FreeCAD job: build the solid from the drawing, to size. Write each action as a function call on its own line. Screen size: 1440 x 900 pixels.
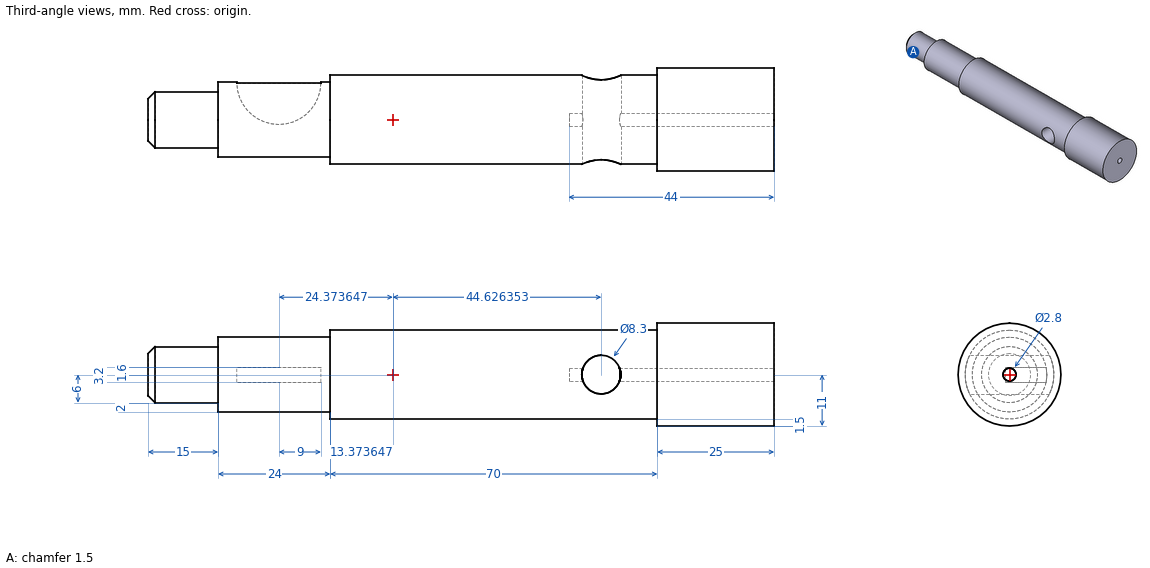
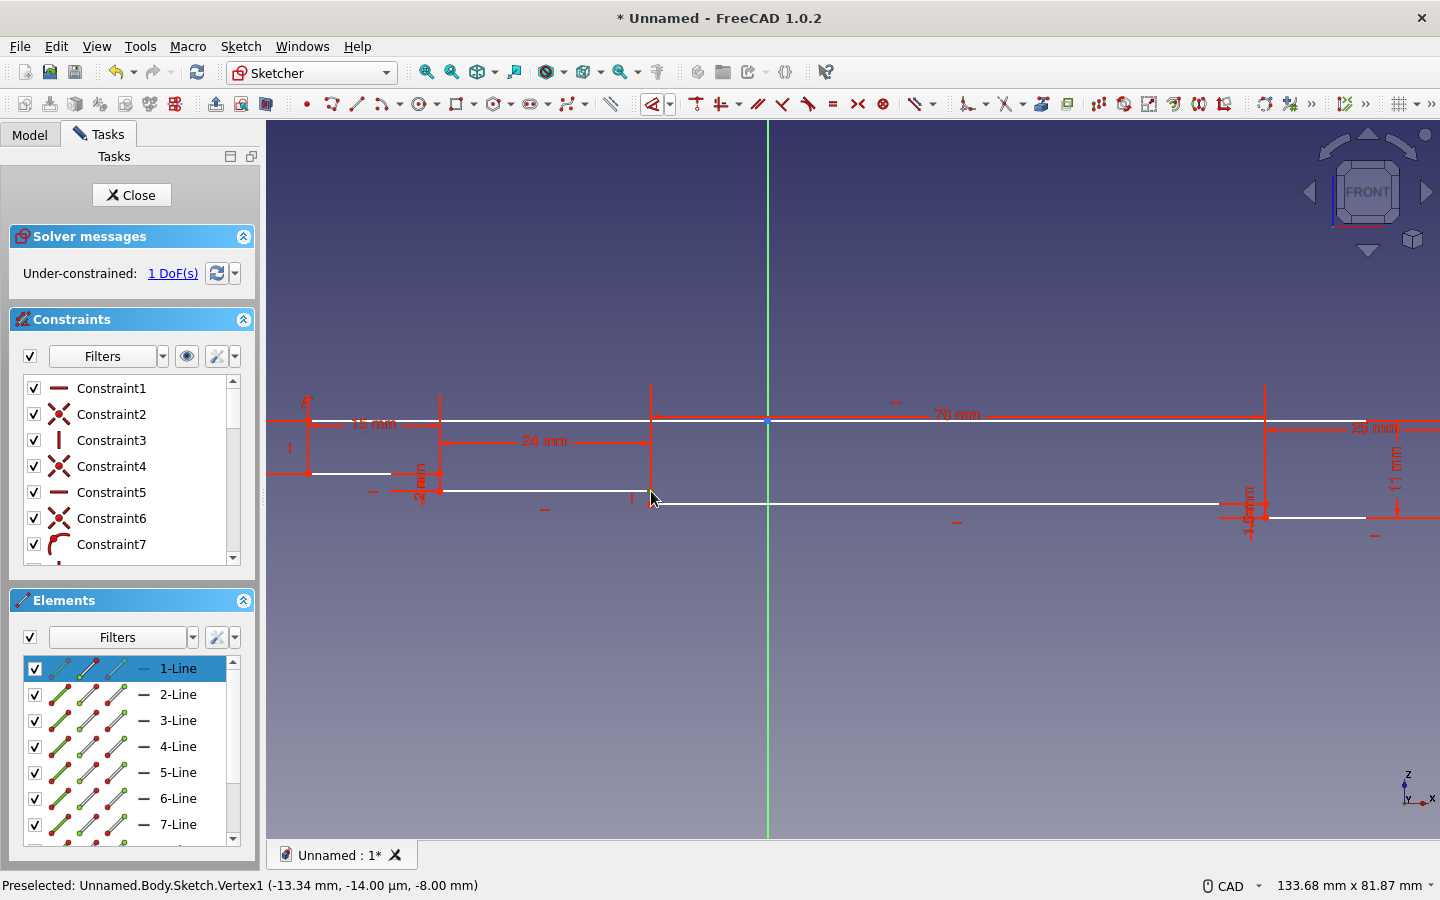
click(670, 104)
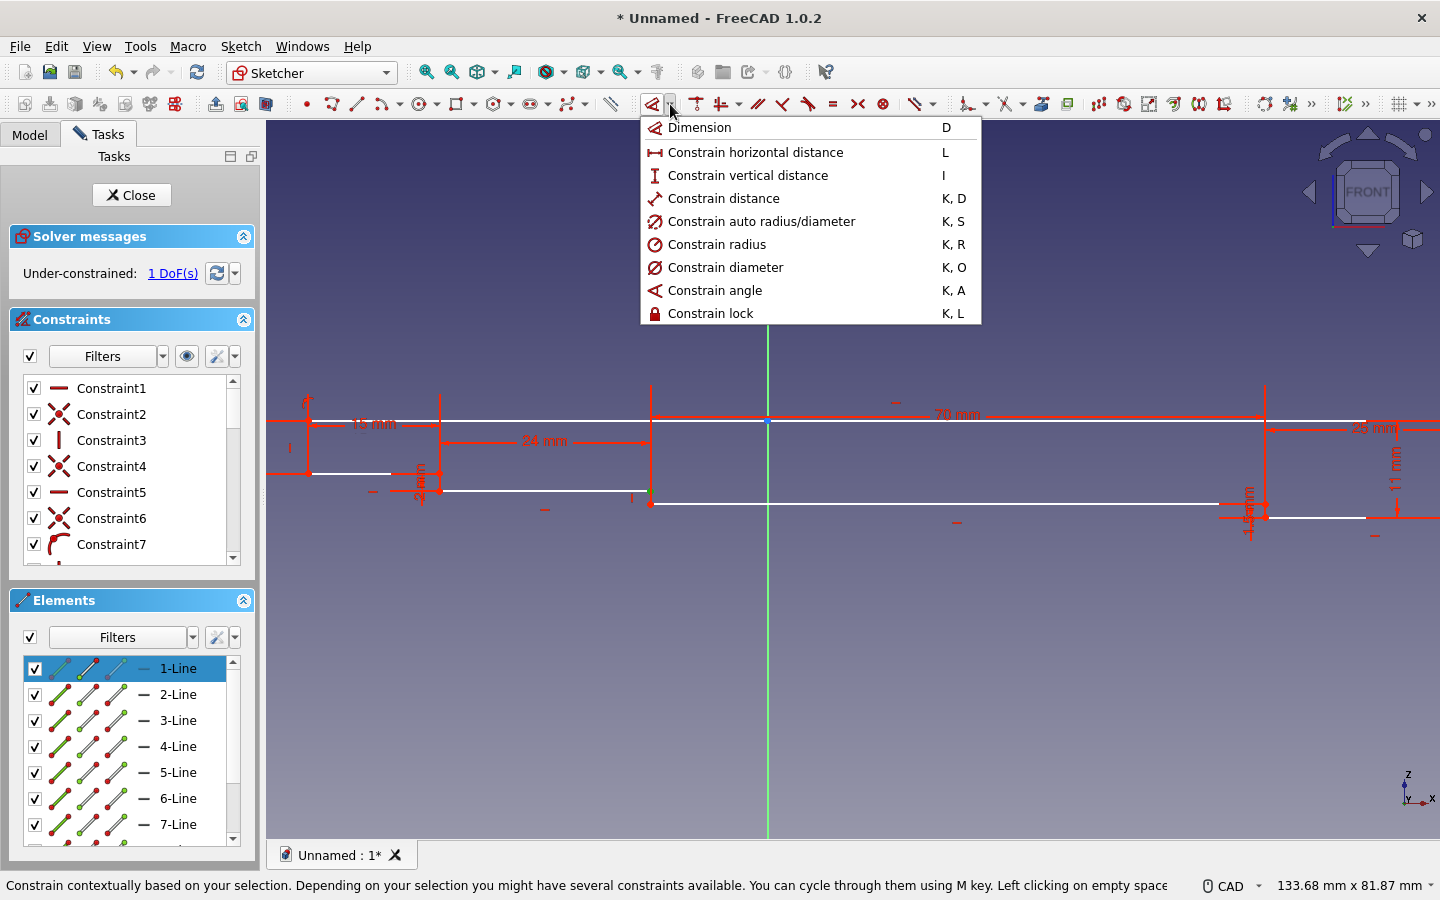
click(811, 152)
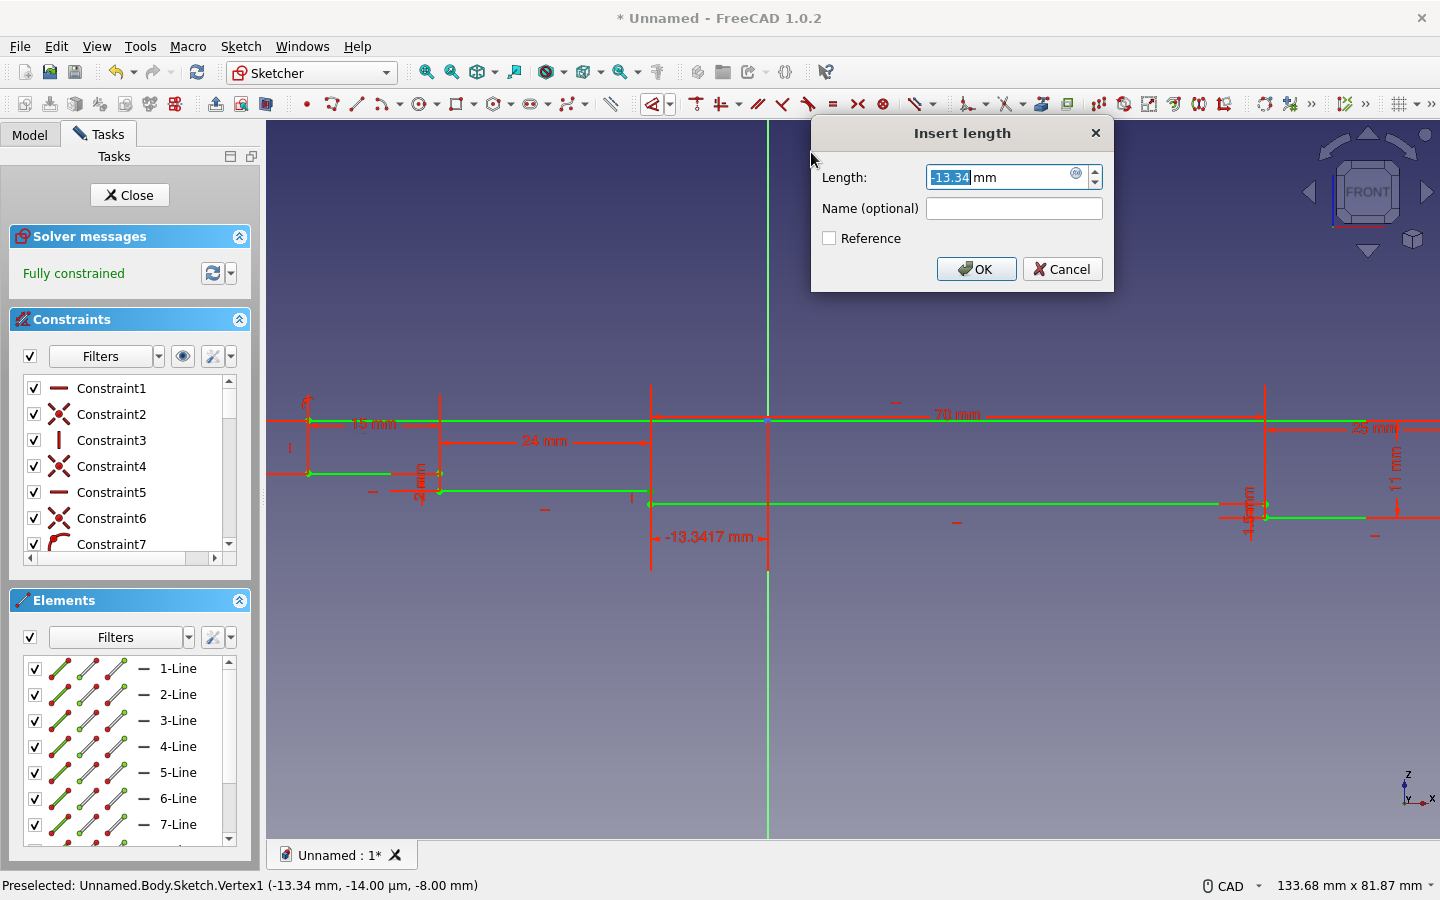
text(-13.373647)
key(Return)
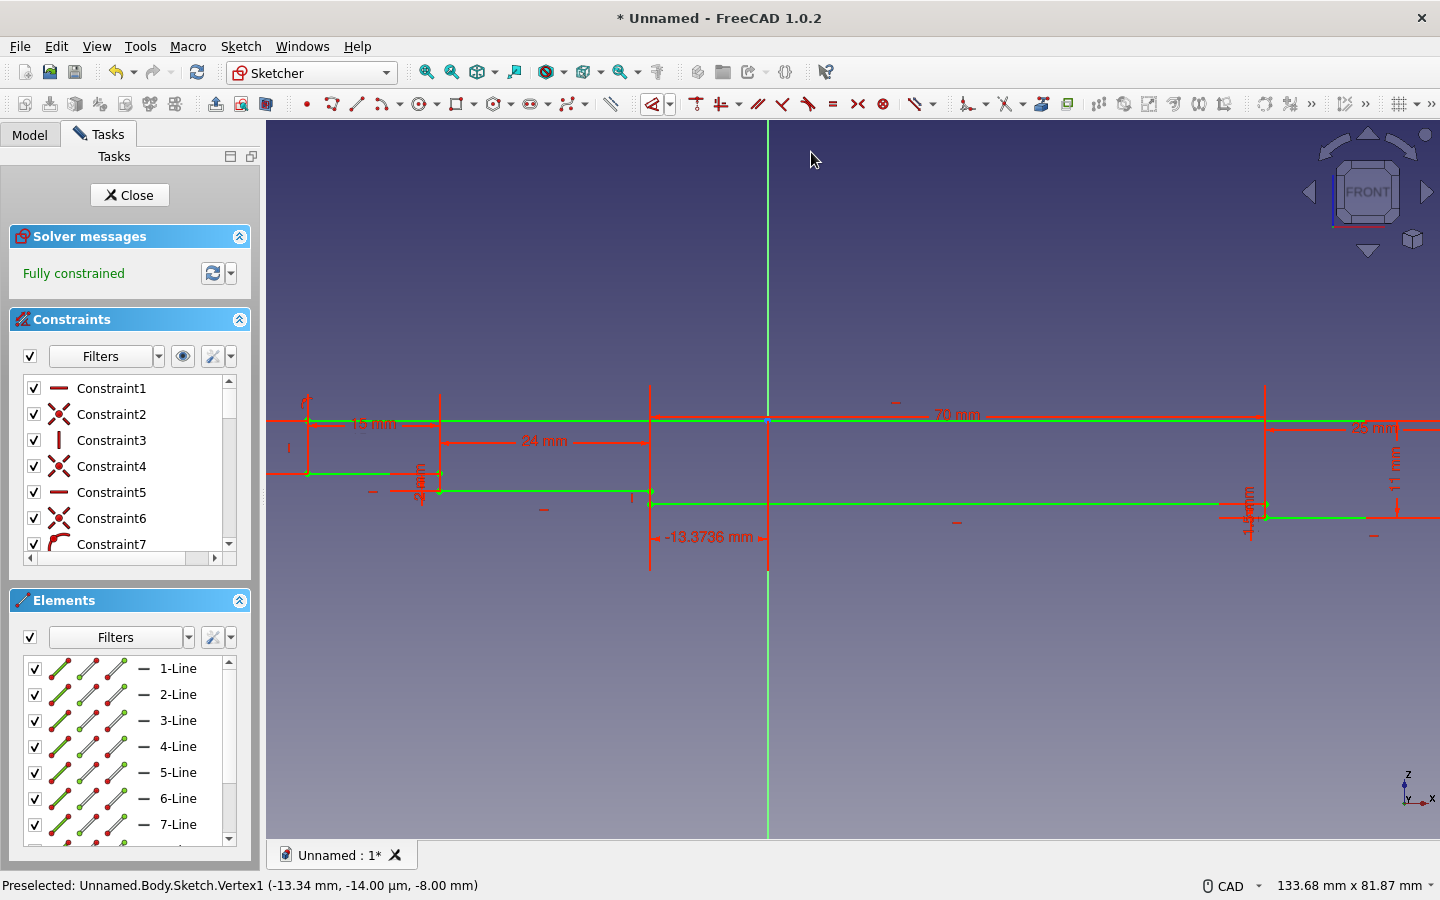
click(130, 195)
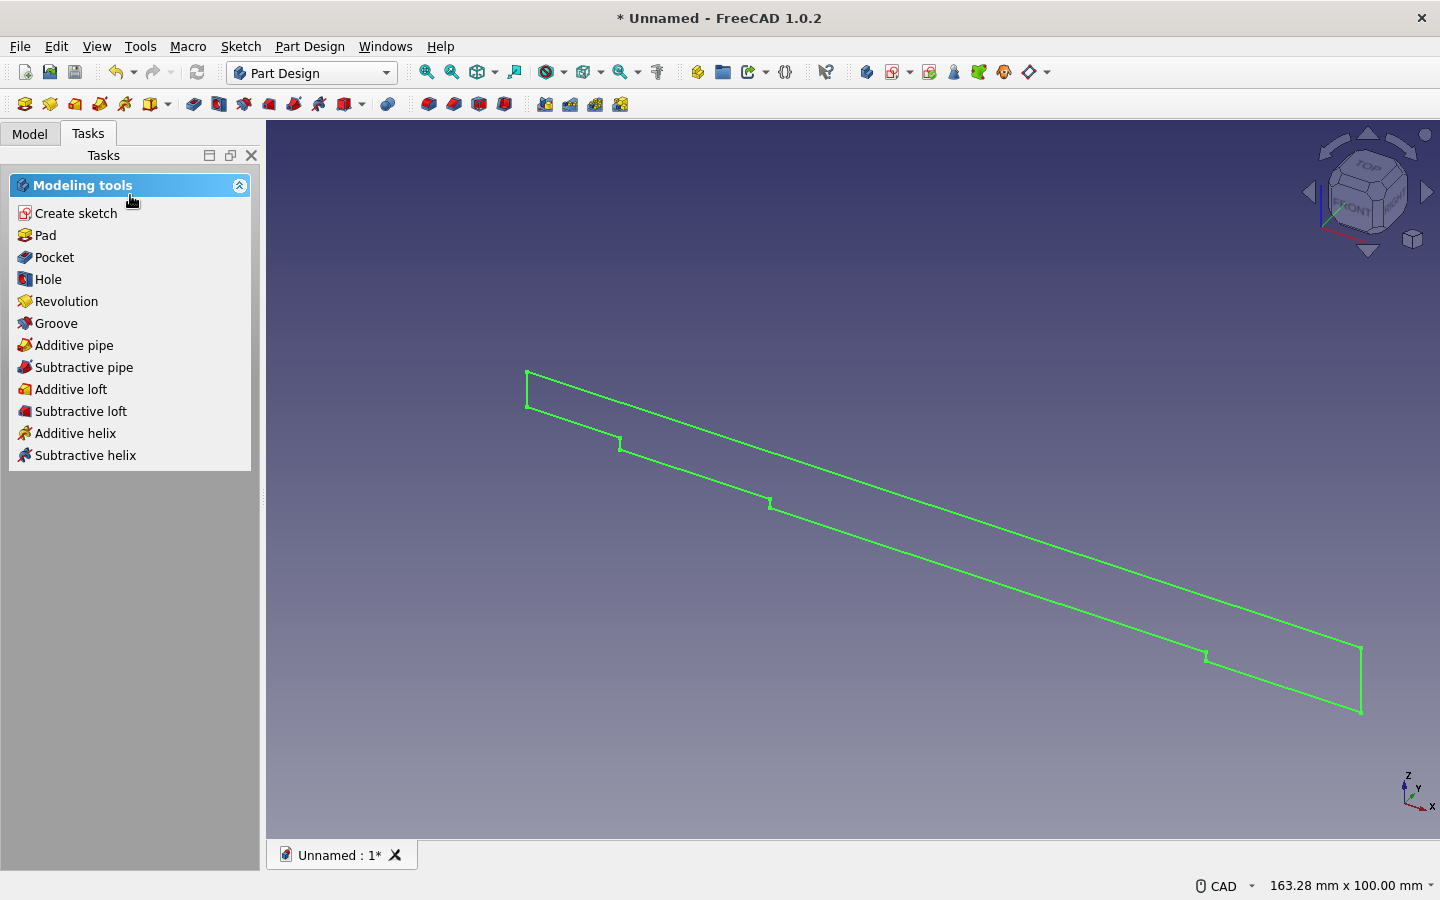
click(50, 104)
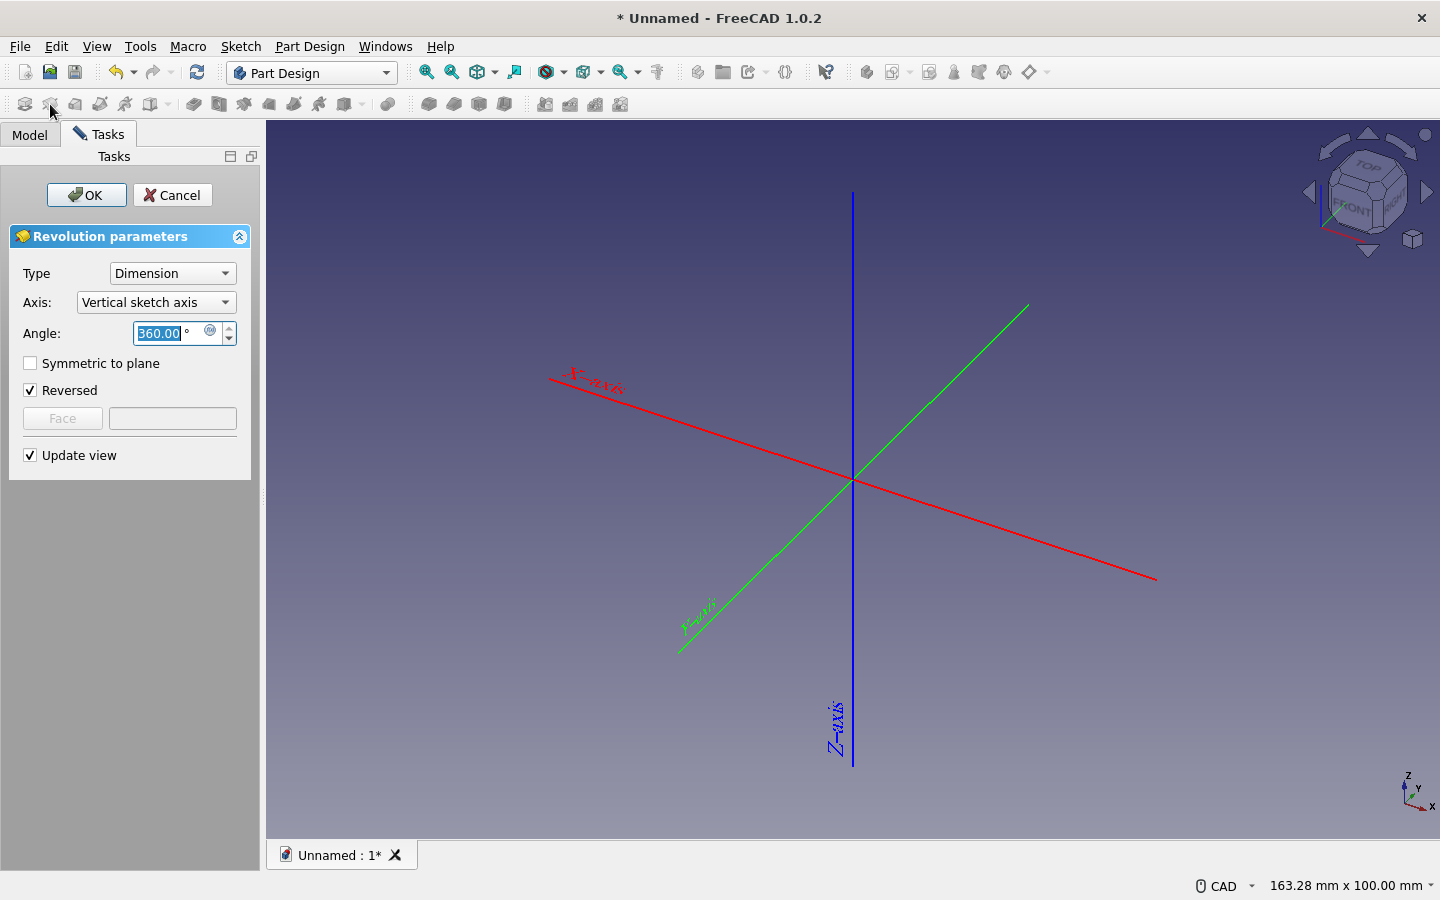
click(157, 302)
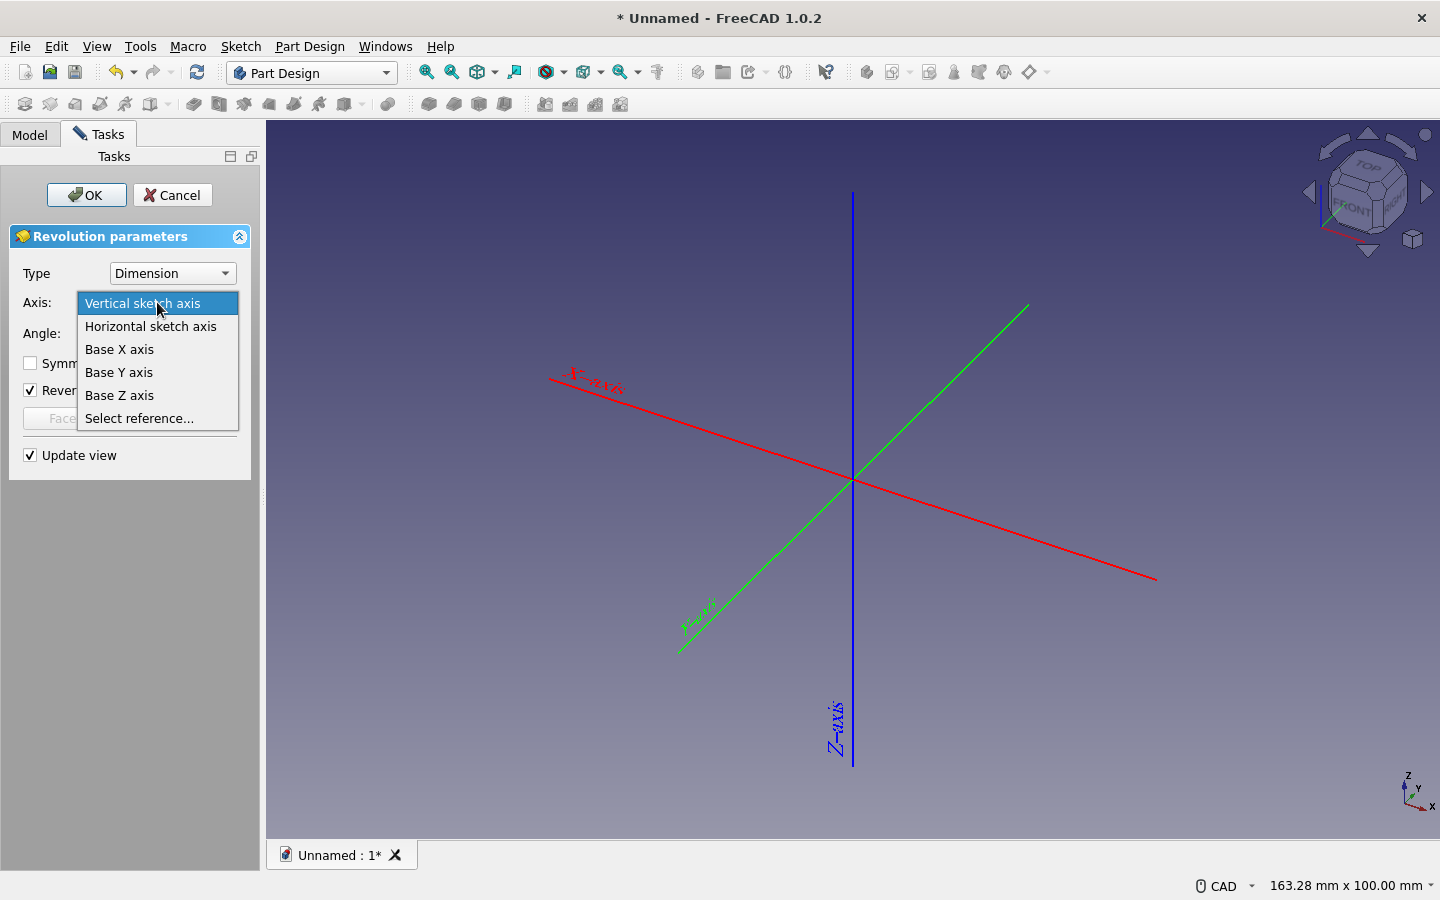
click(156, 326)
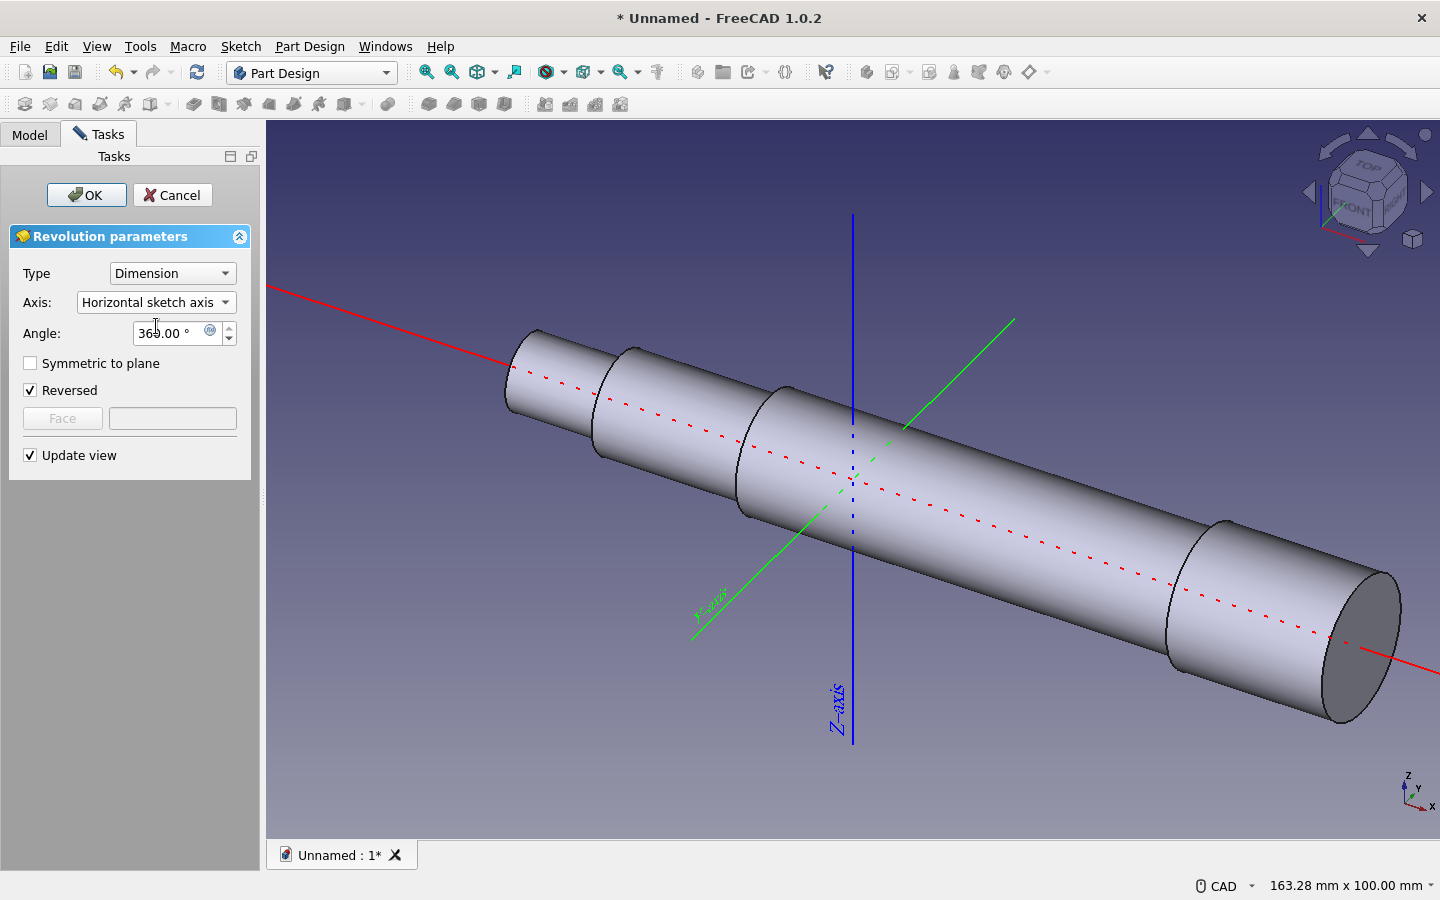
click(87, 195)